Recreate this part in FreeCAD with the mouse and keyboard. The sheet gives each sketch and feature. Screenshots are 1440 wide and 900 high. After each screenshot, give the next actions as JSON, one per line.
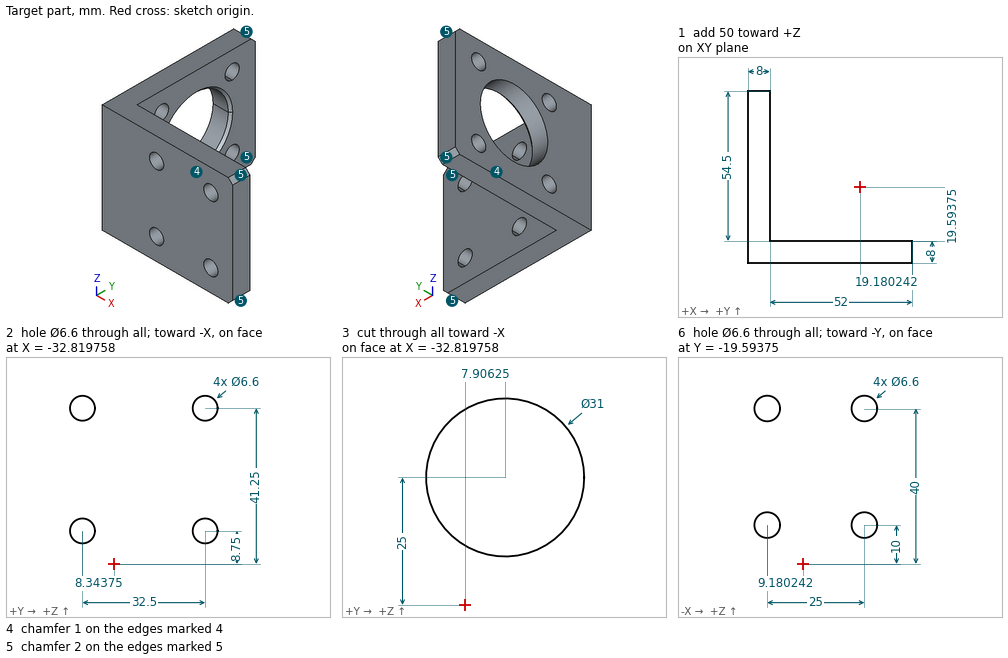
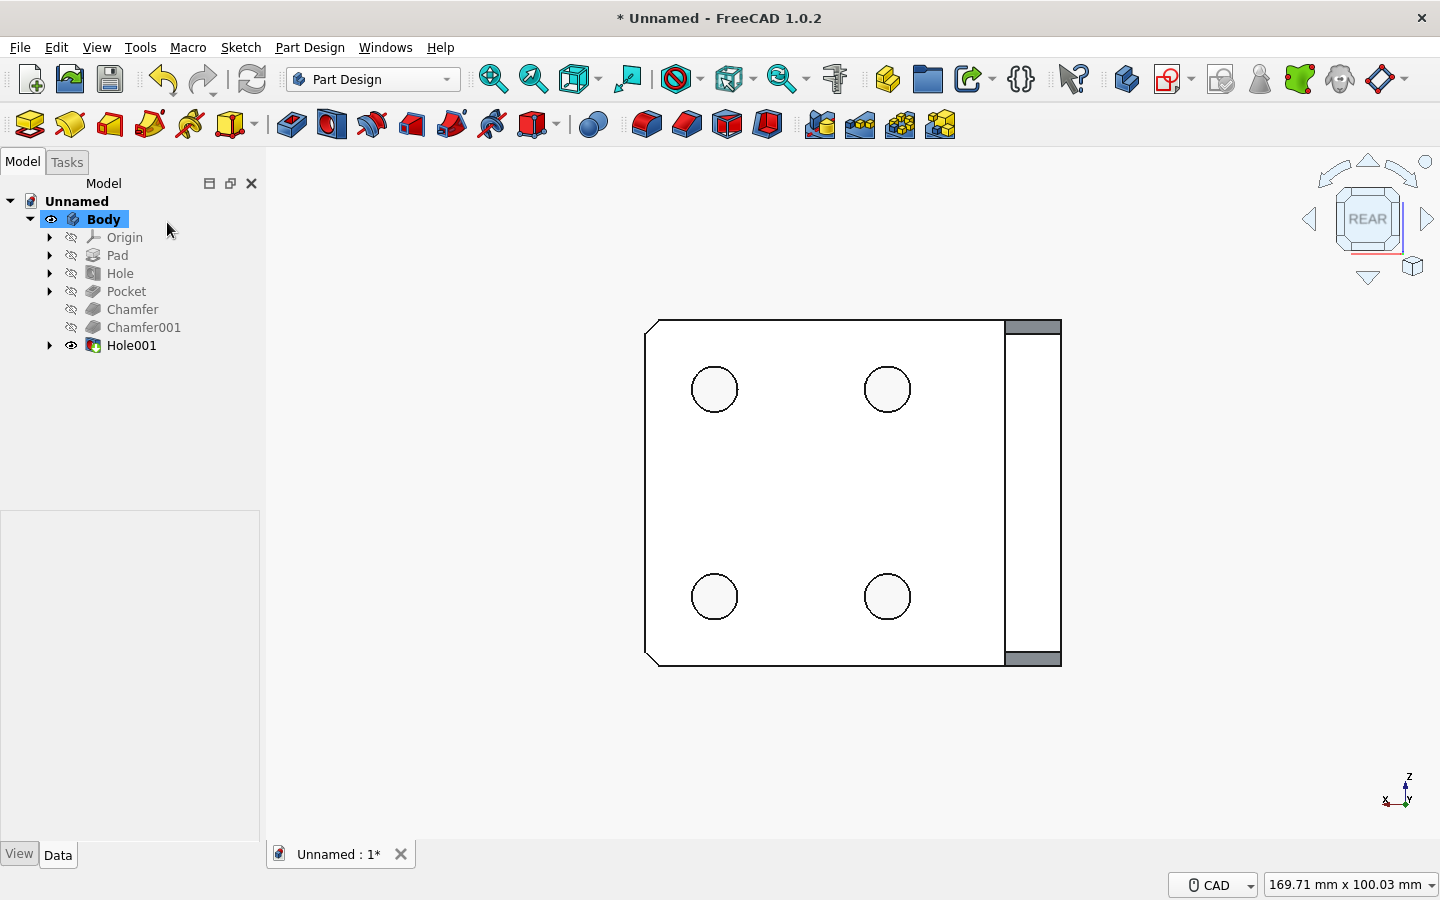
{"action": "key", "text": "0"}